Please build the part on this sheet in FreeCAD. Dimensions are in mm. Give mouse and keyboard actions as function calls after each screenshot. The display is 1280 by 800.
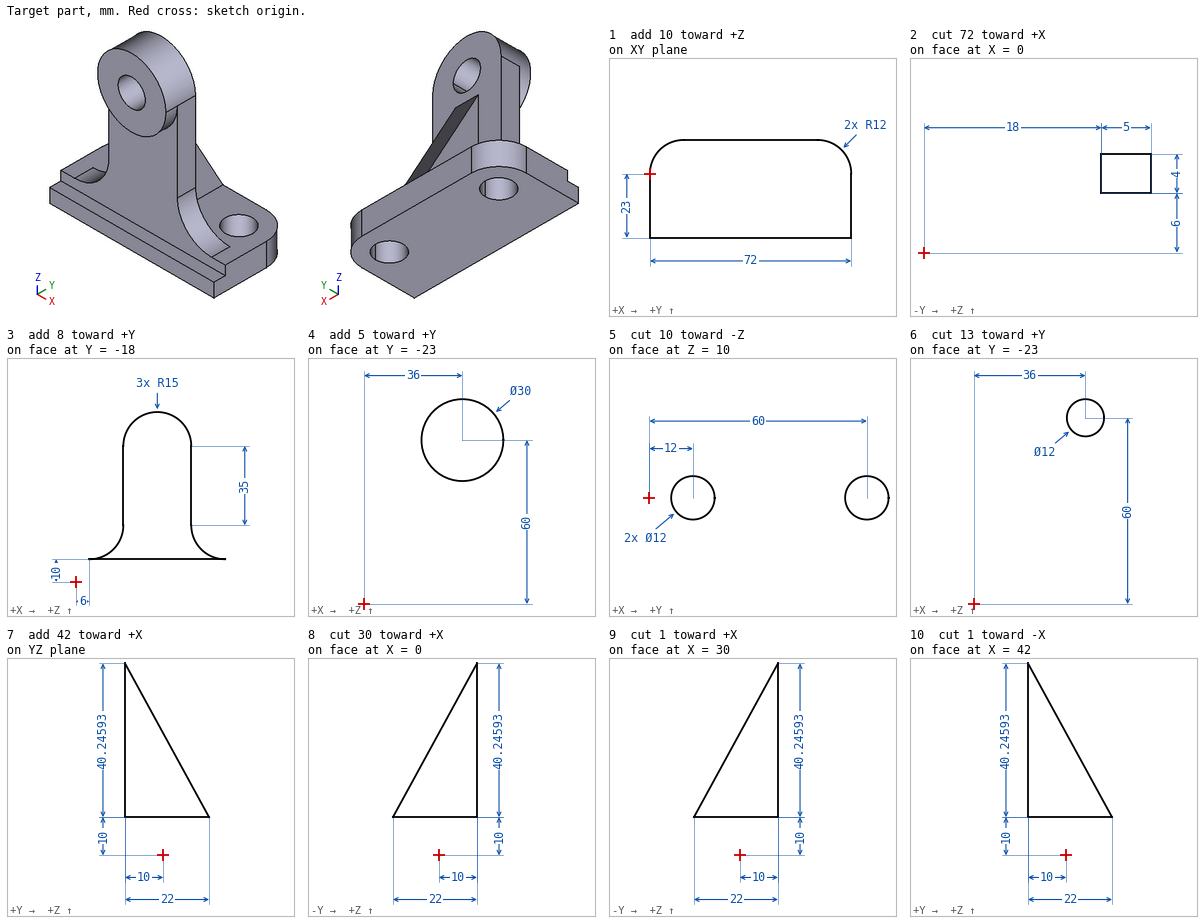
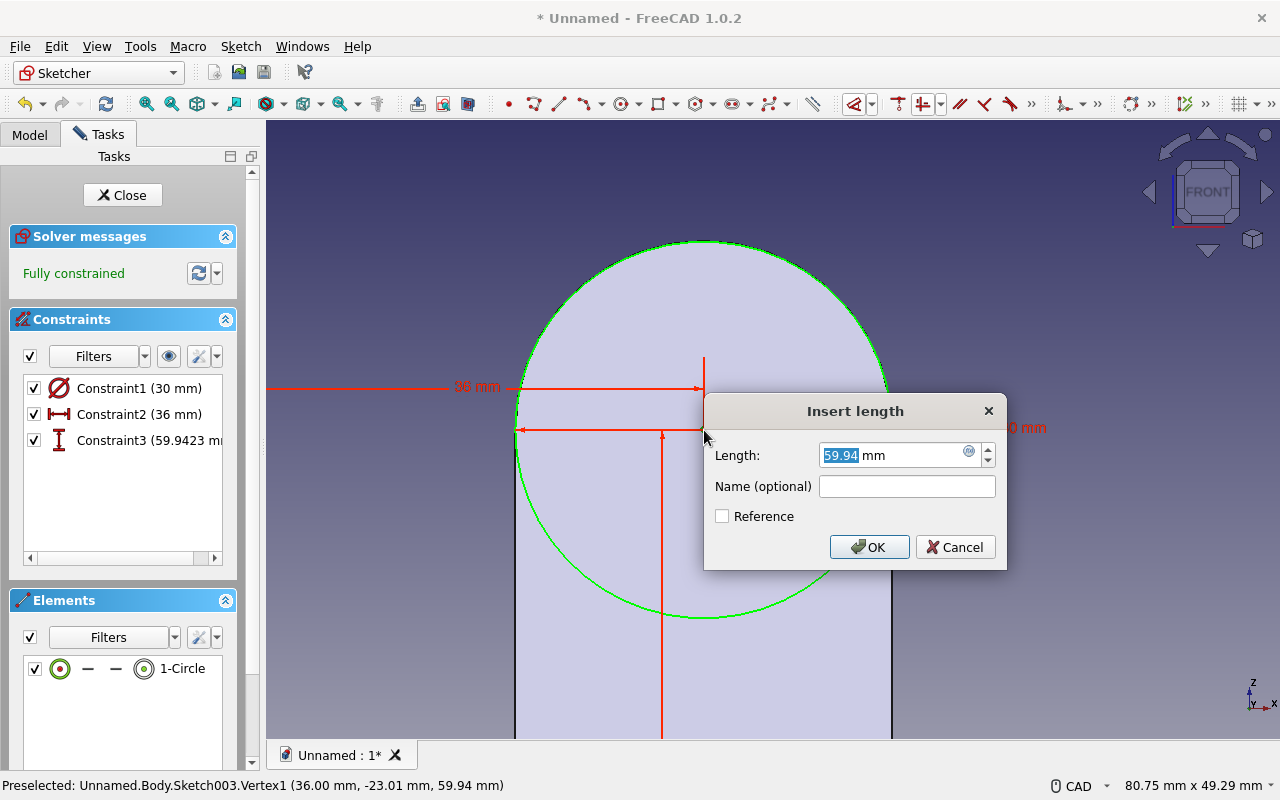
text(60)
key(Return)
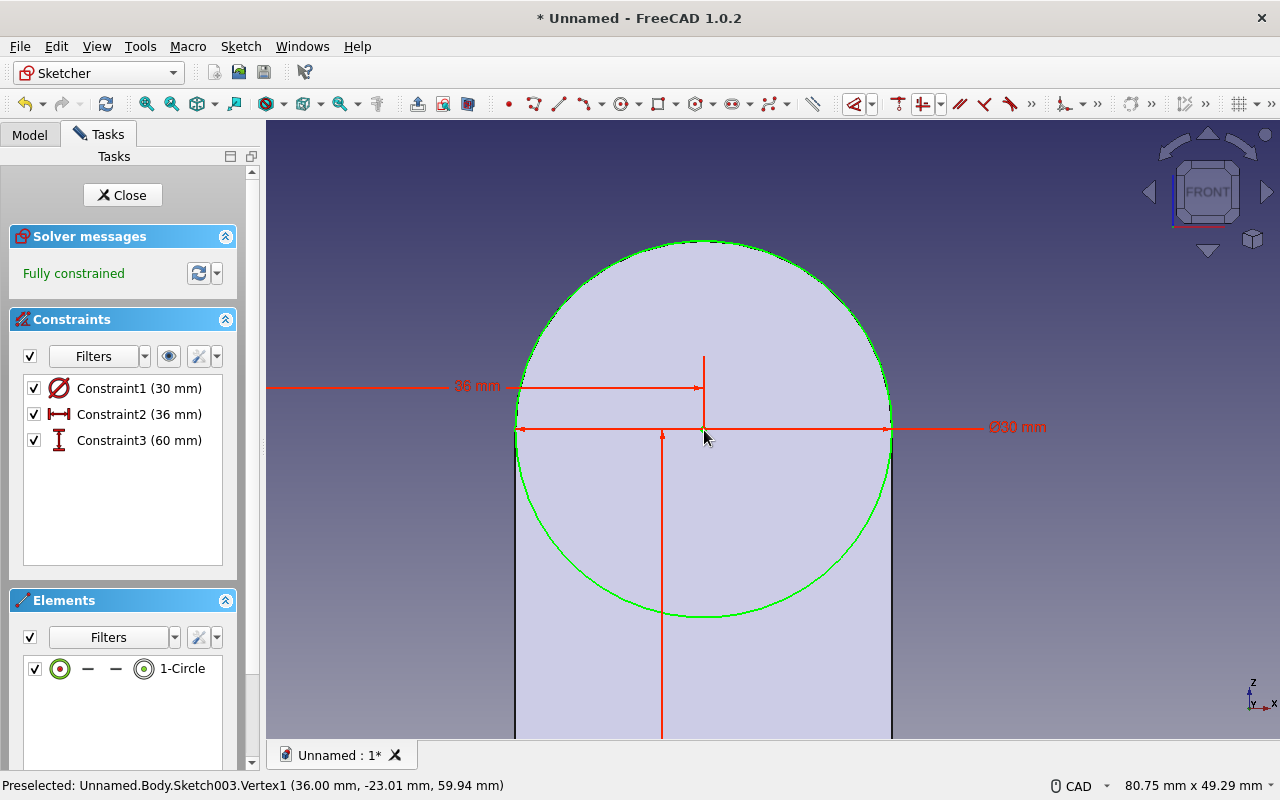
click(123, 195)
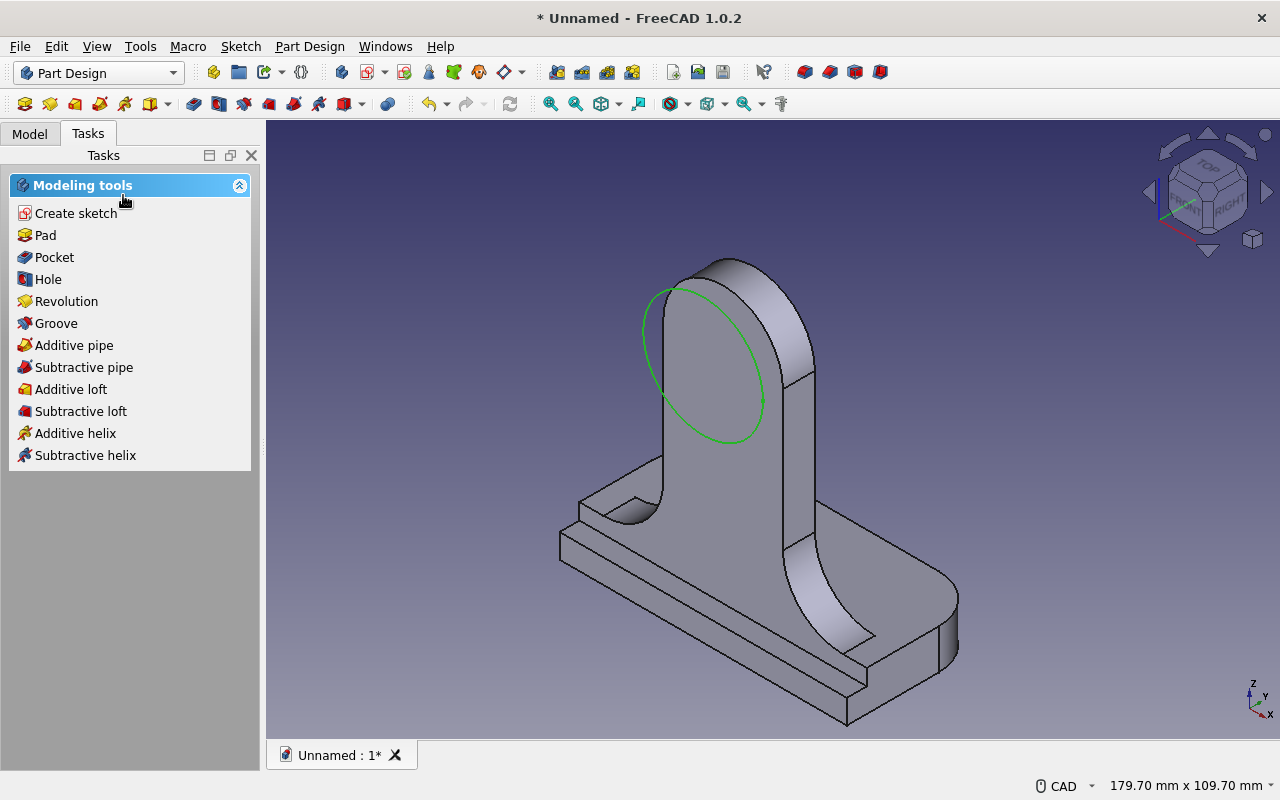
click(25, 104)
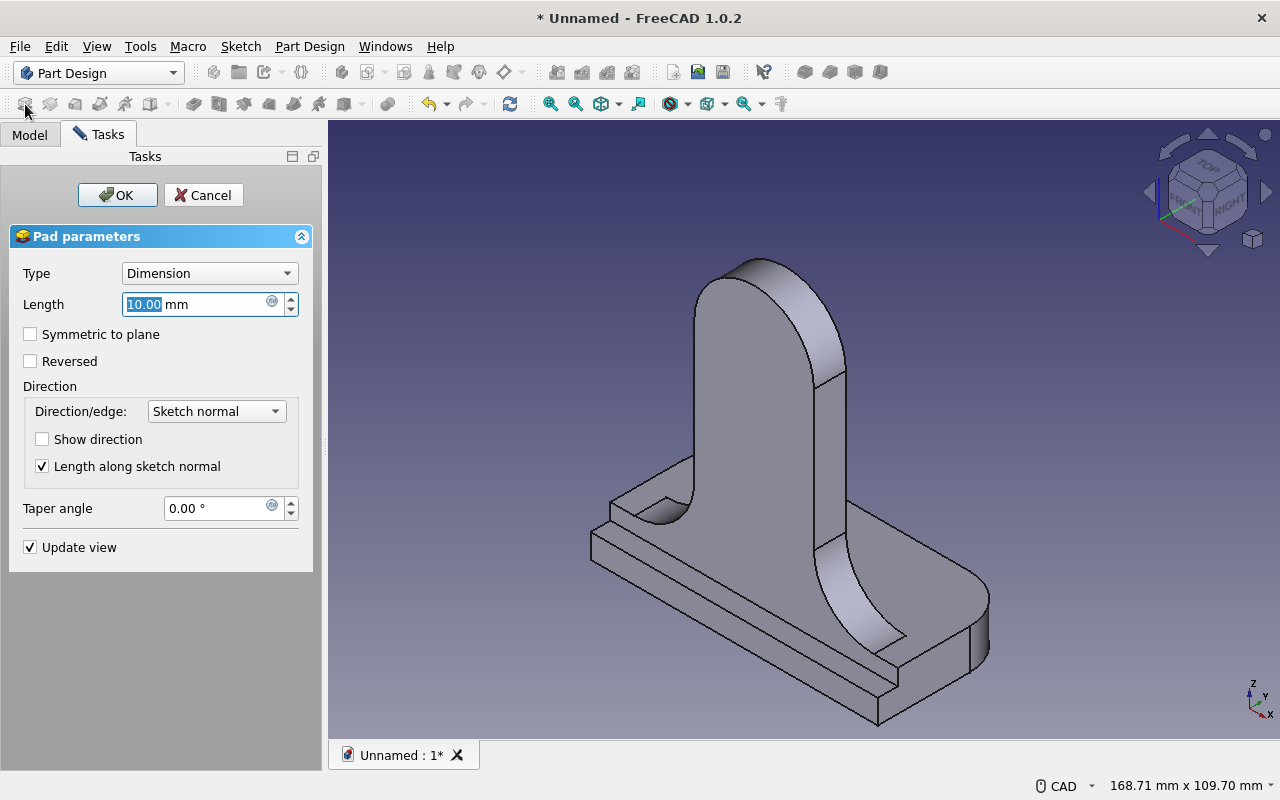
text(5)
key(Tab)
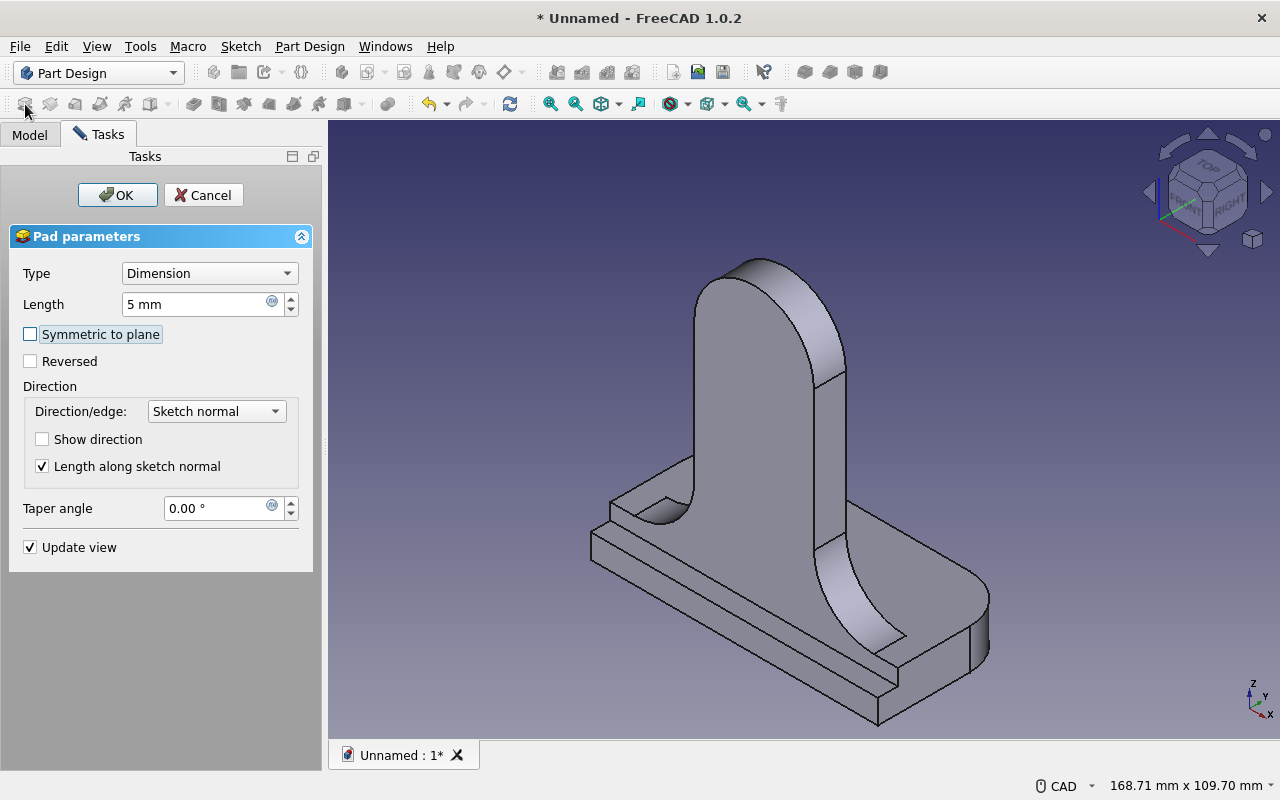
click(31, 361)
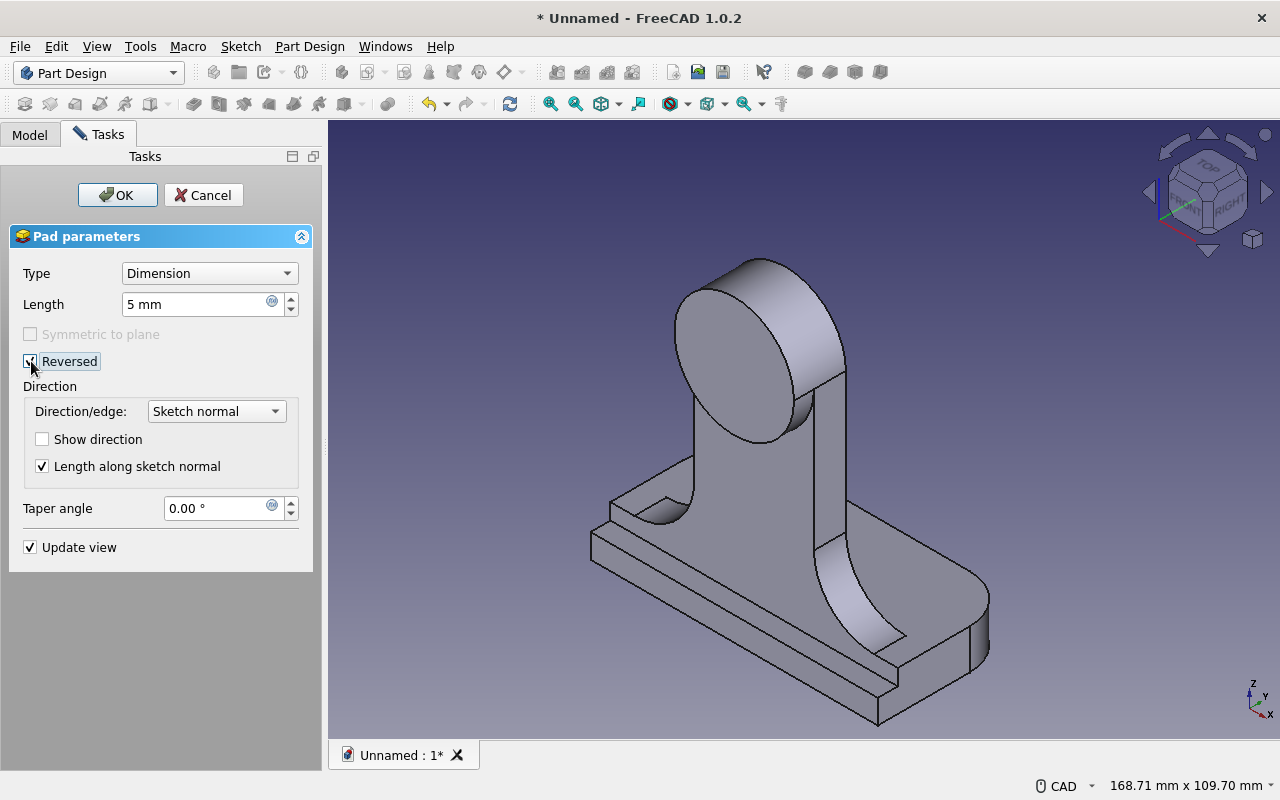
click(118, 195)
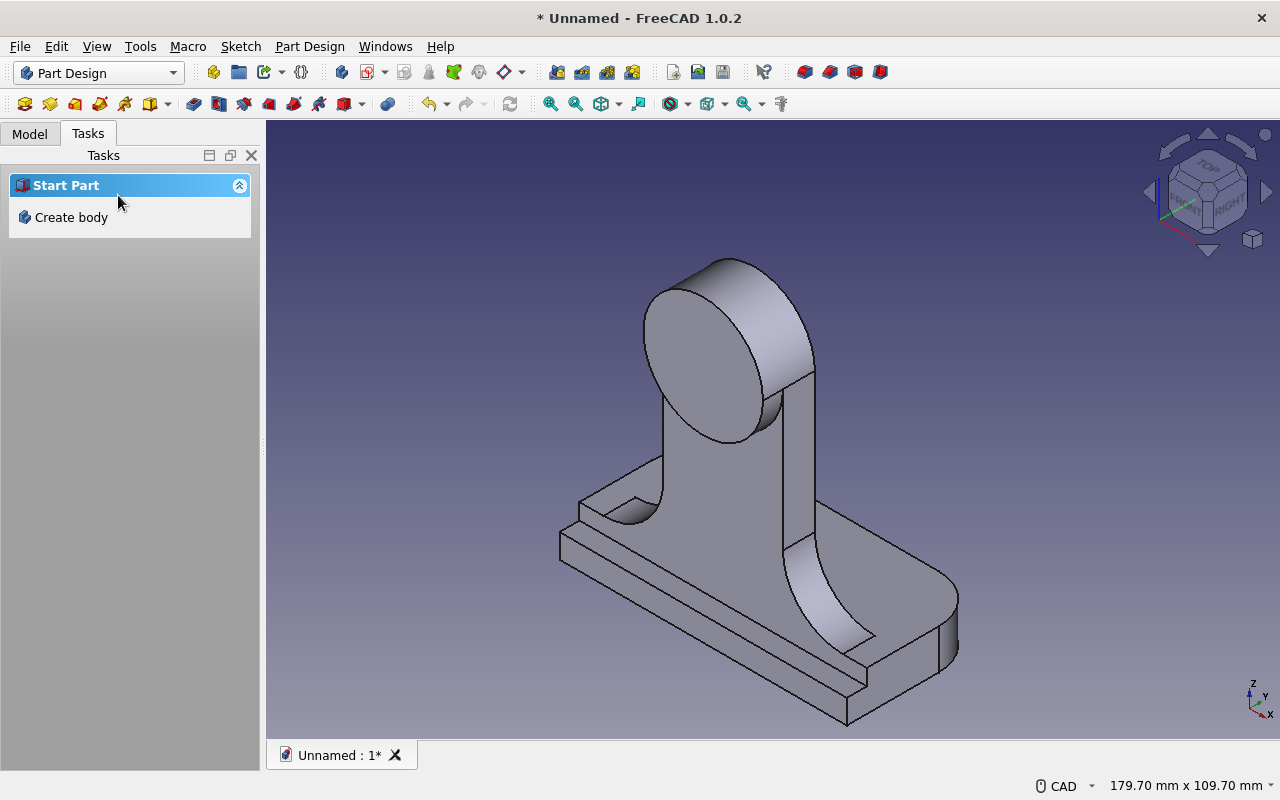
click(882, 587)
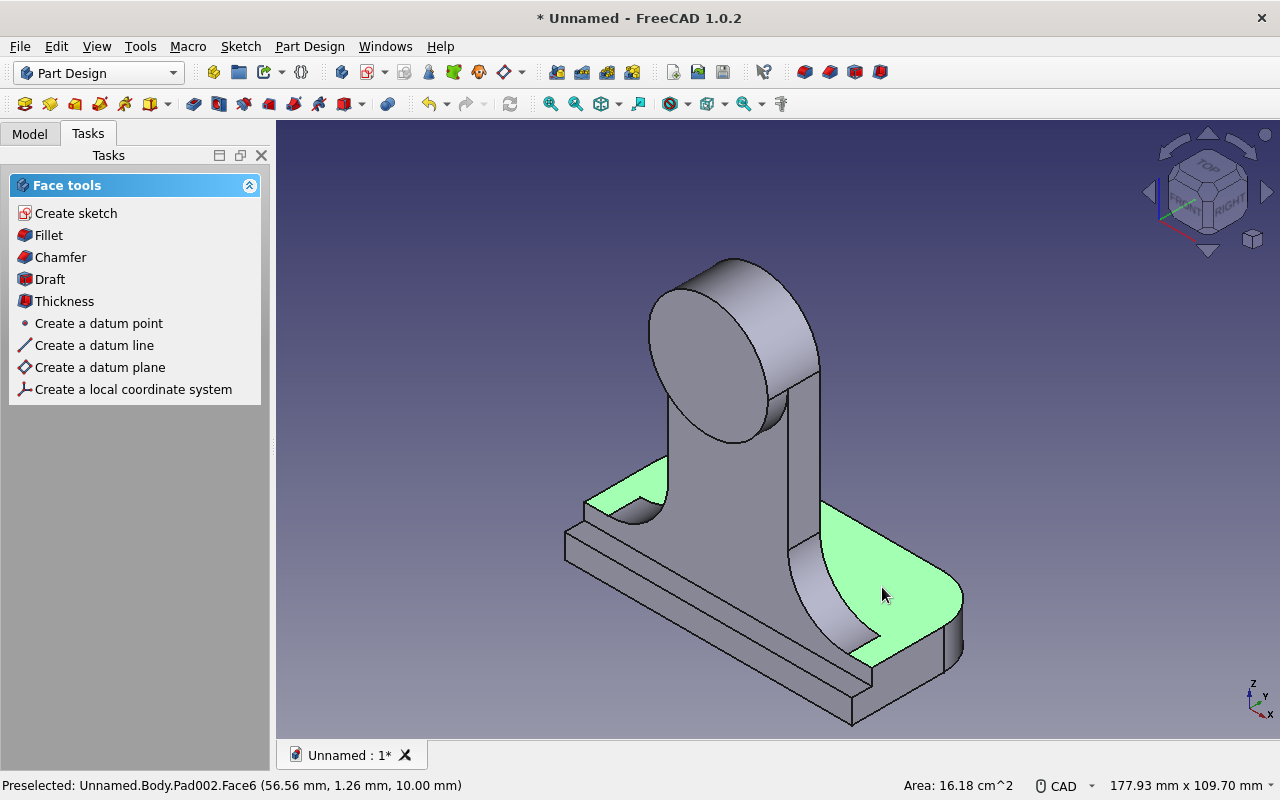
click(366, 72)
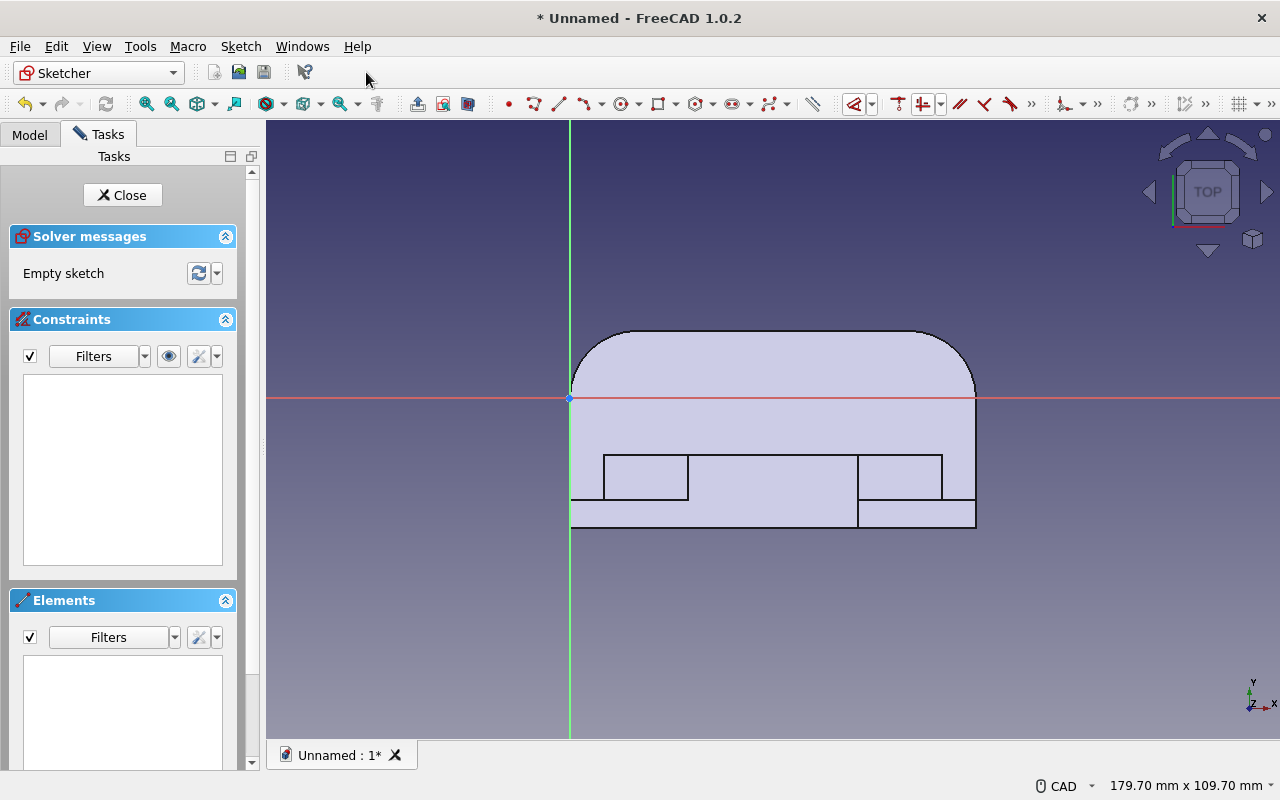
key(q)
key(s)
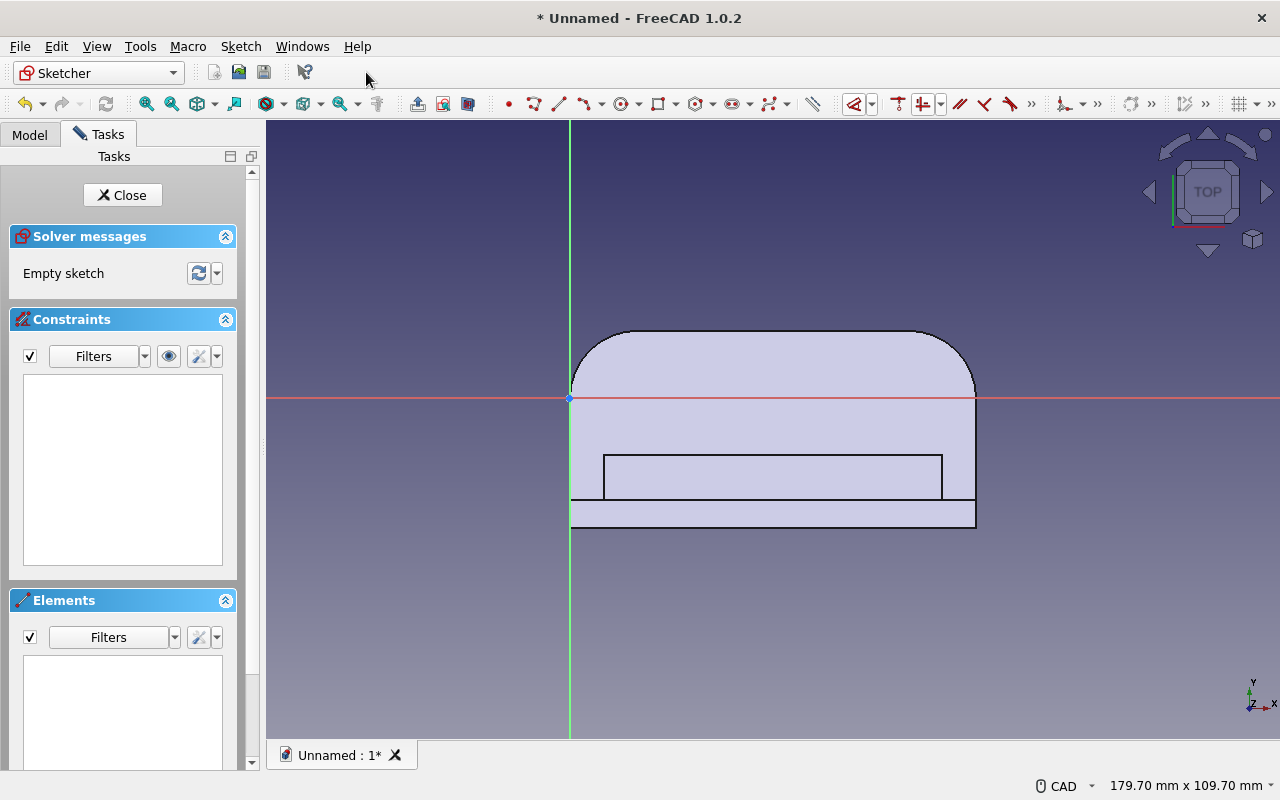
scroll(861, 335, up, 2)